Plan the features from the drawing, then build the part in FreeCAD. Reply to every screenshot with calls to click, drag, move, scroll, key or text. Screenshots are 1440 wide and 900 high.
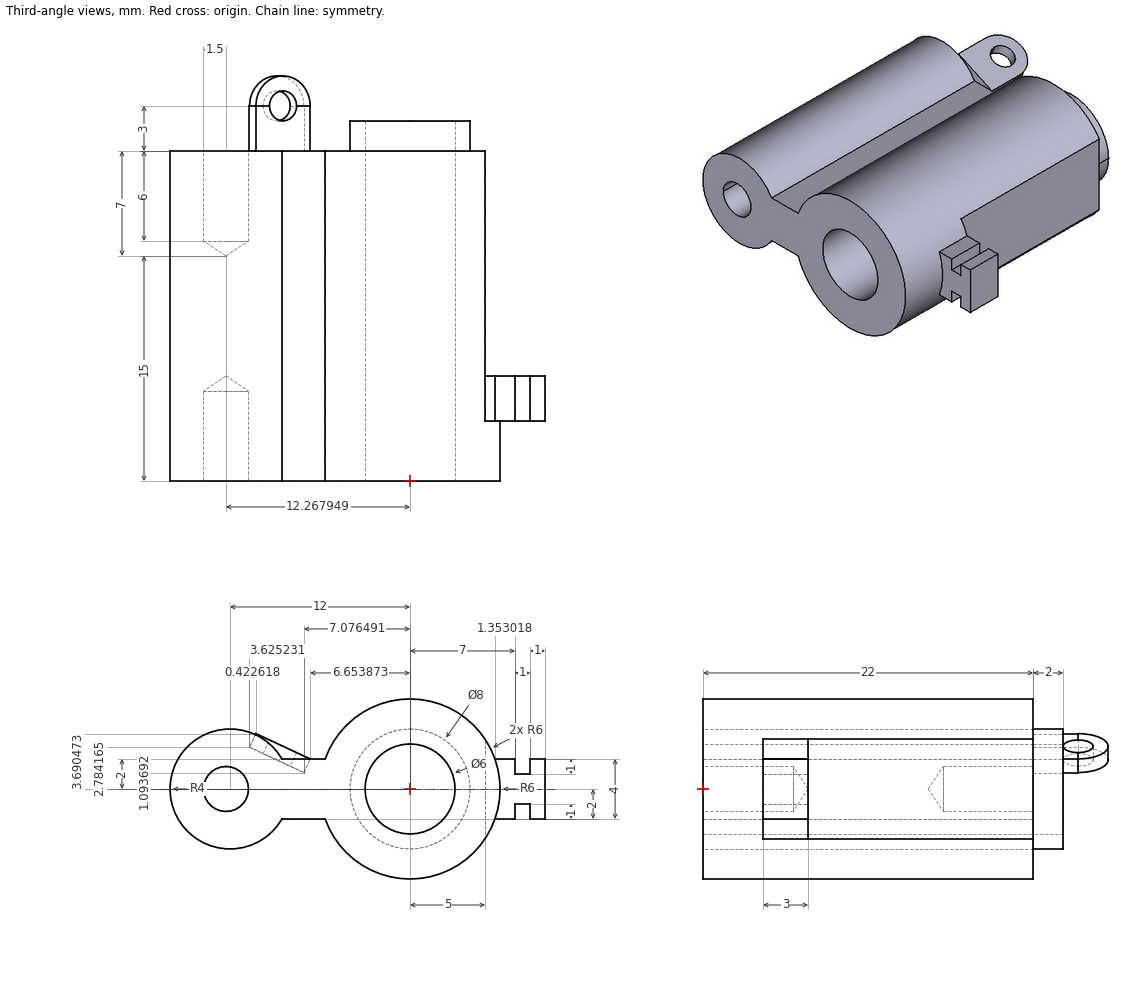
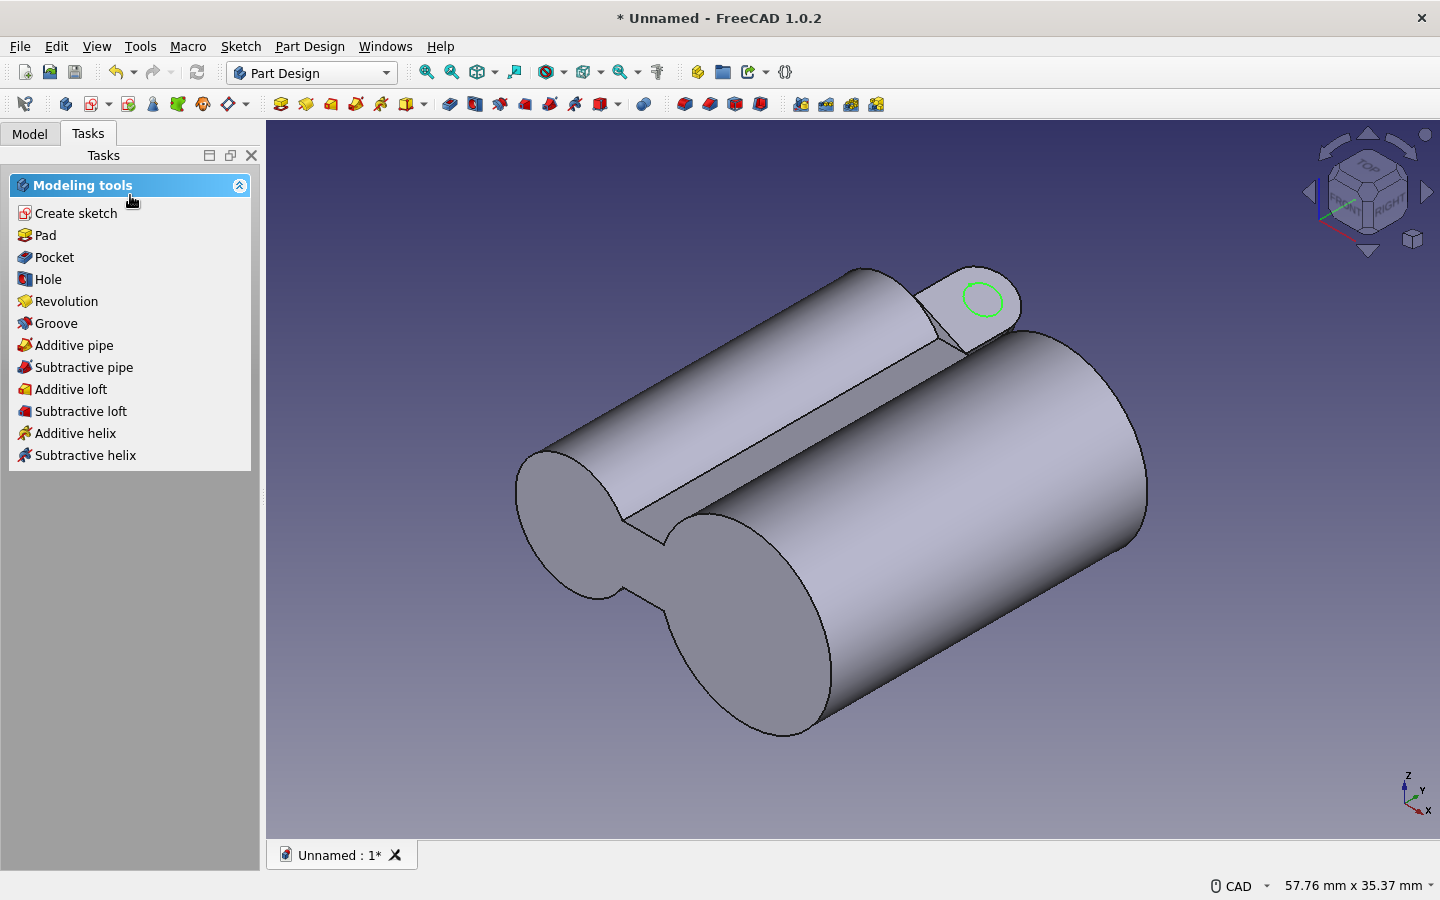
click(450, 104)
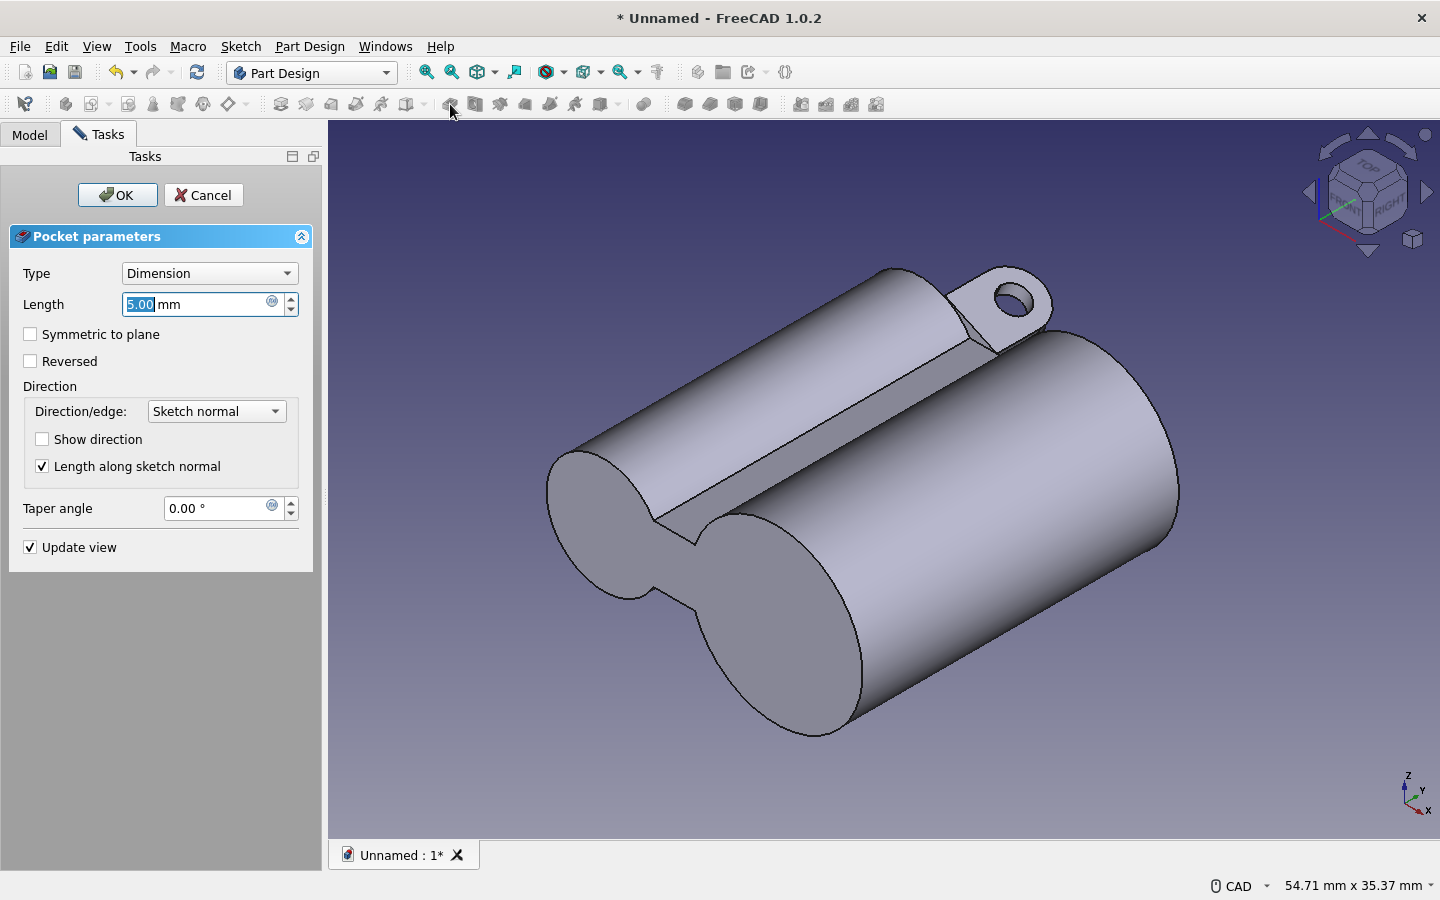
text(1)
key(Tab)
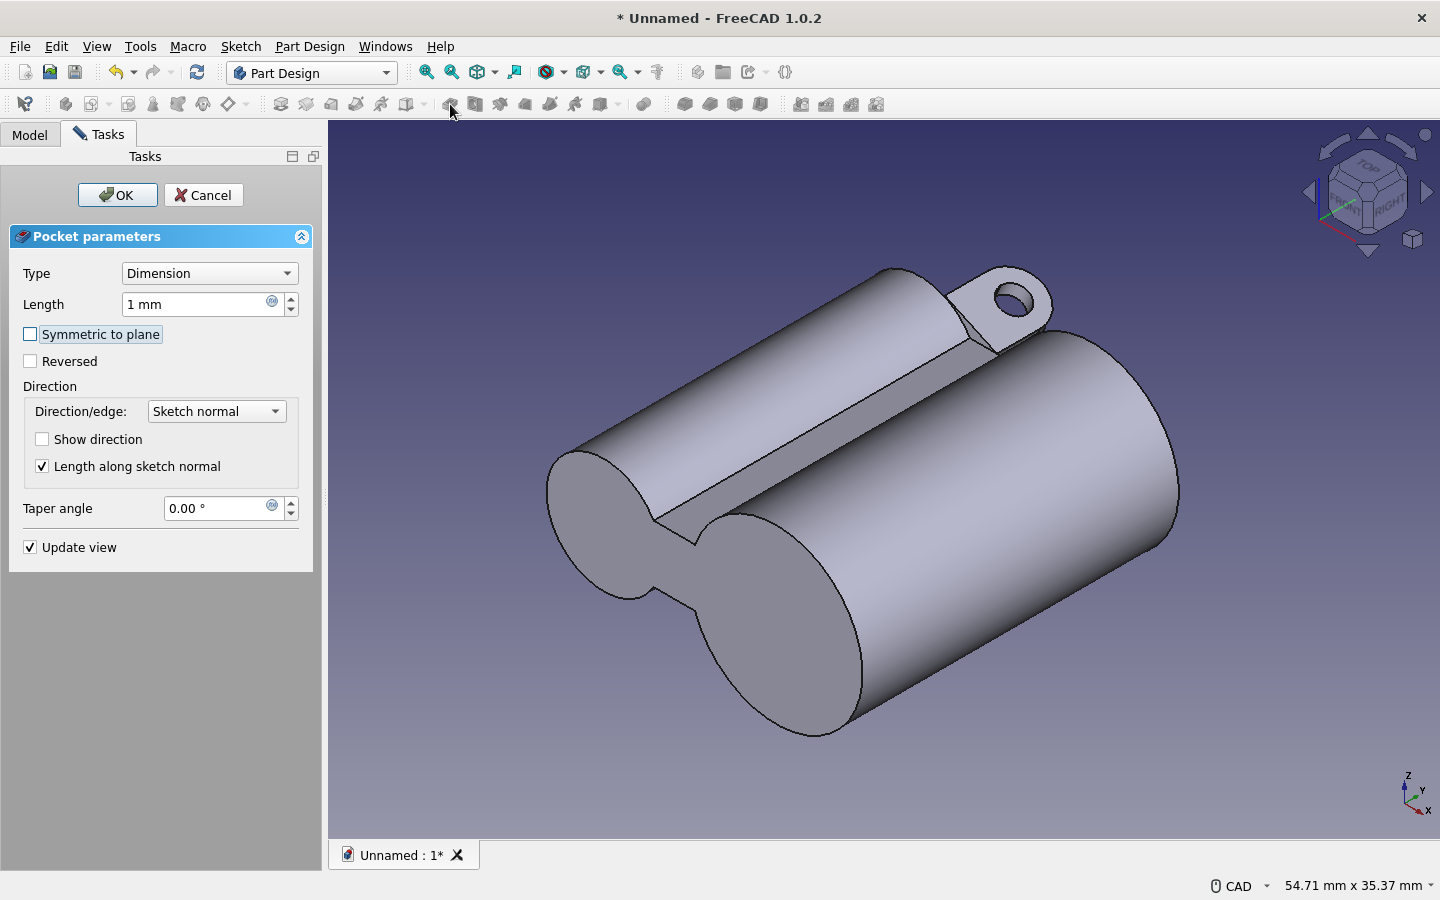
click(118, 195)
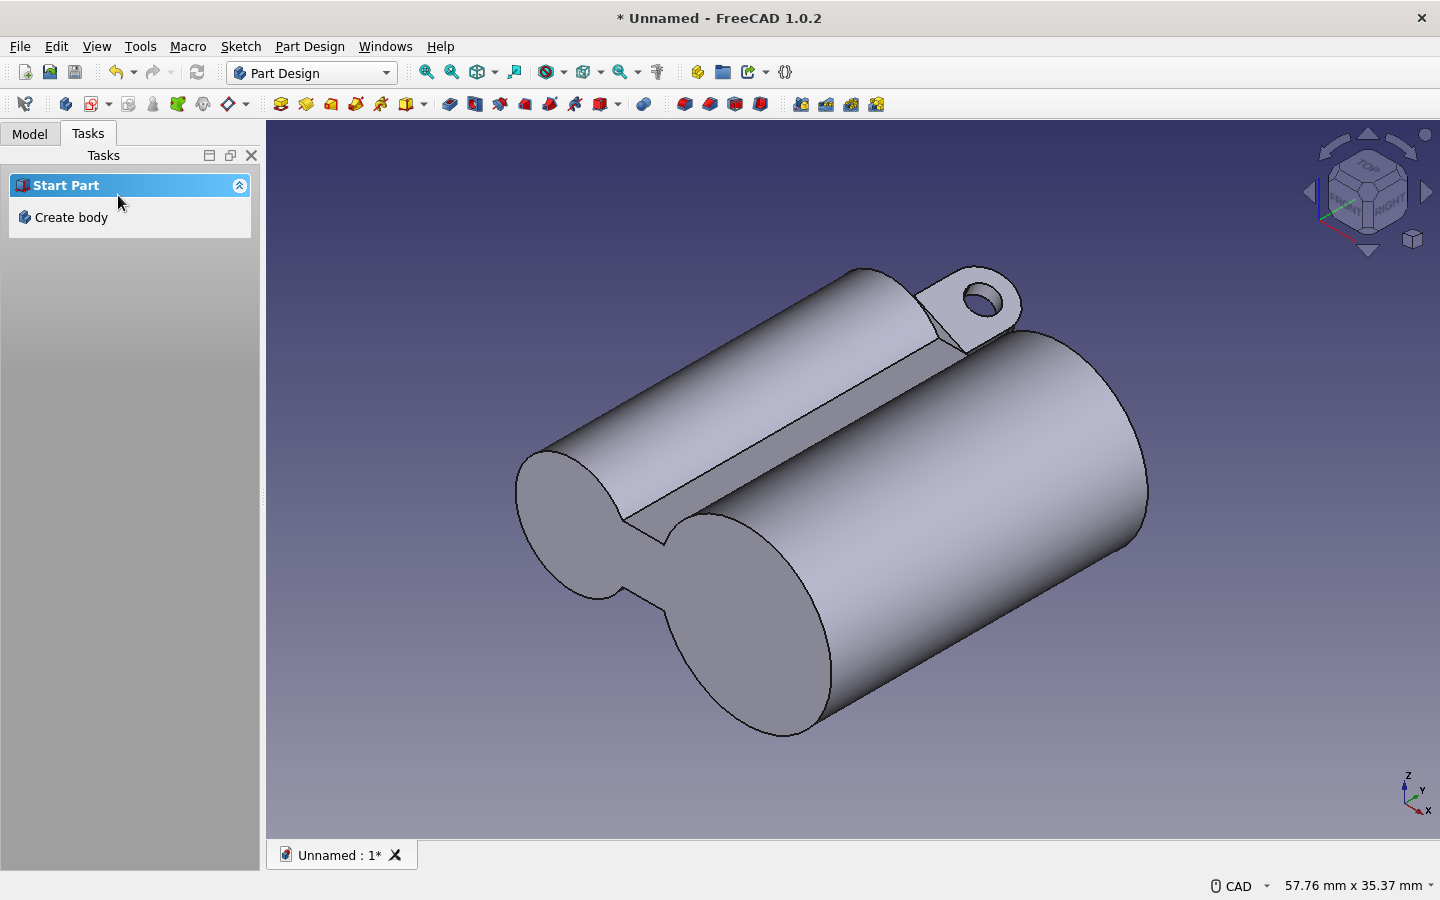
click(90, 104)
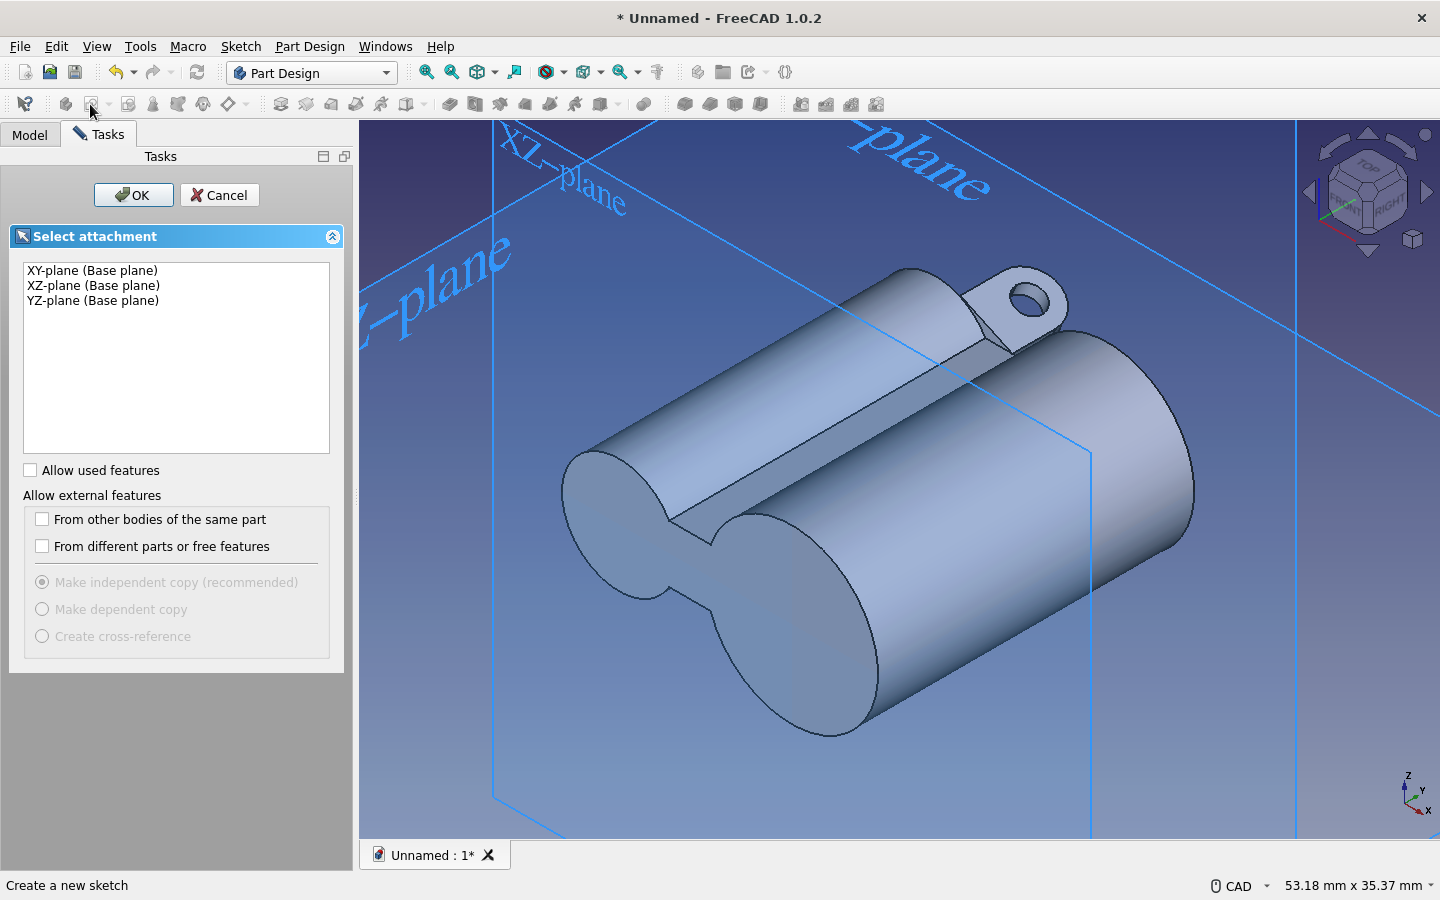
click(84, 270)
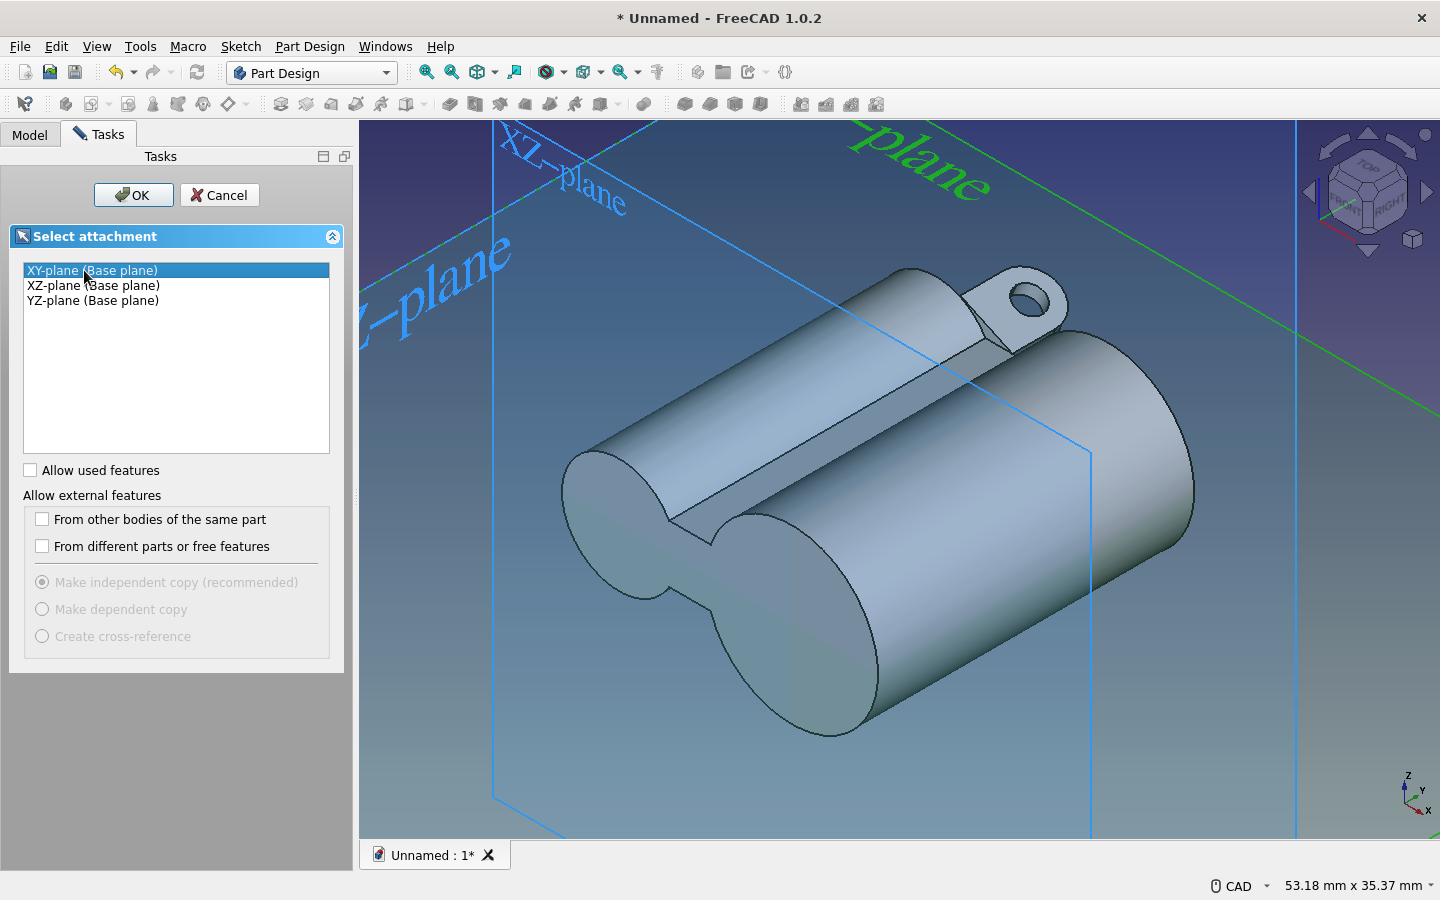
click(134, 195)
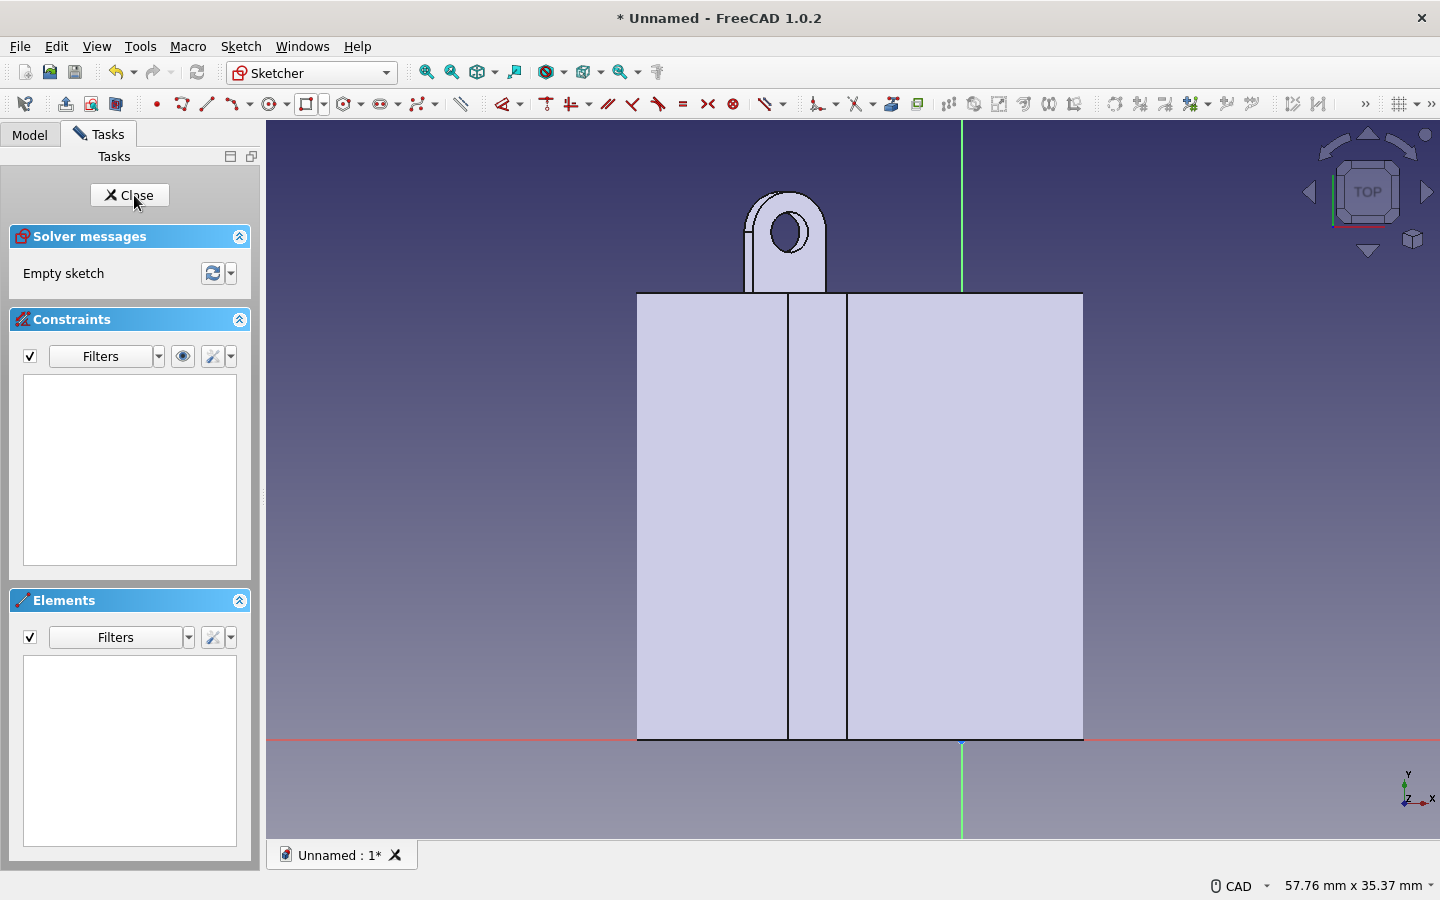
click(116, 104)